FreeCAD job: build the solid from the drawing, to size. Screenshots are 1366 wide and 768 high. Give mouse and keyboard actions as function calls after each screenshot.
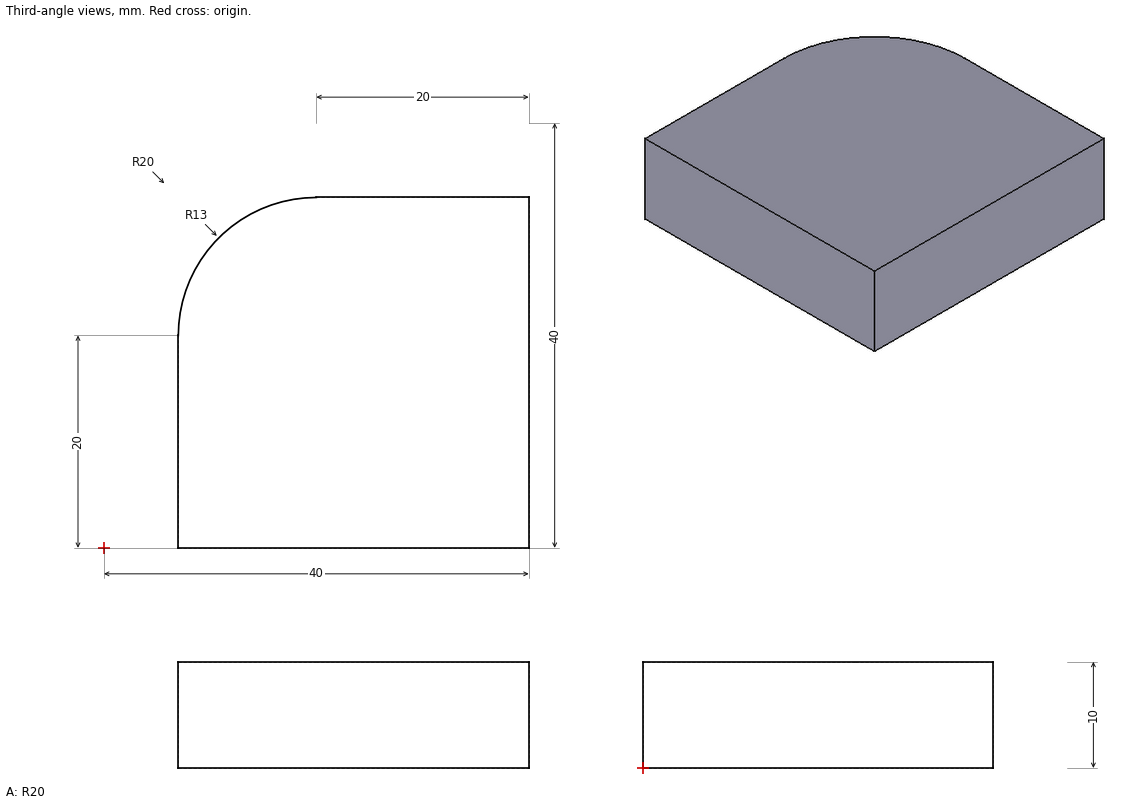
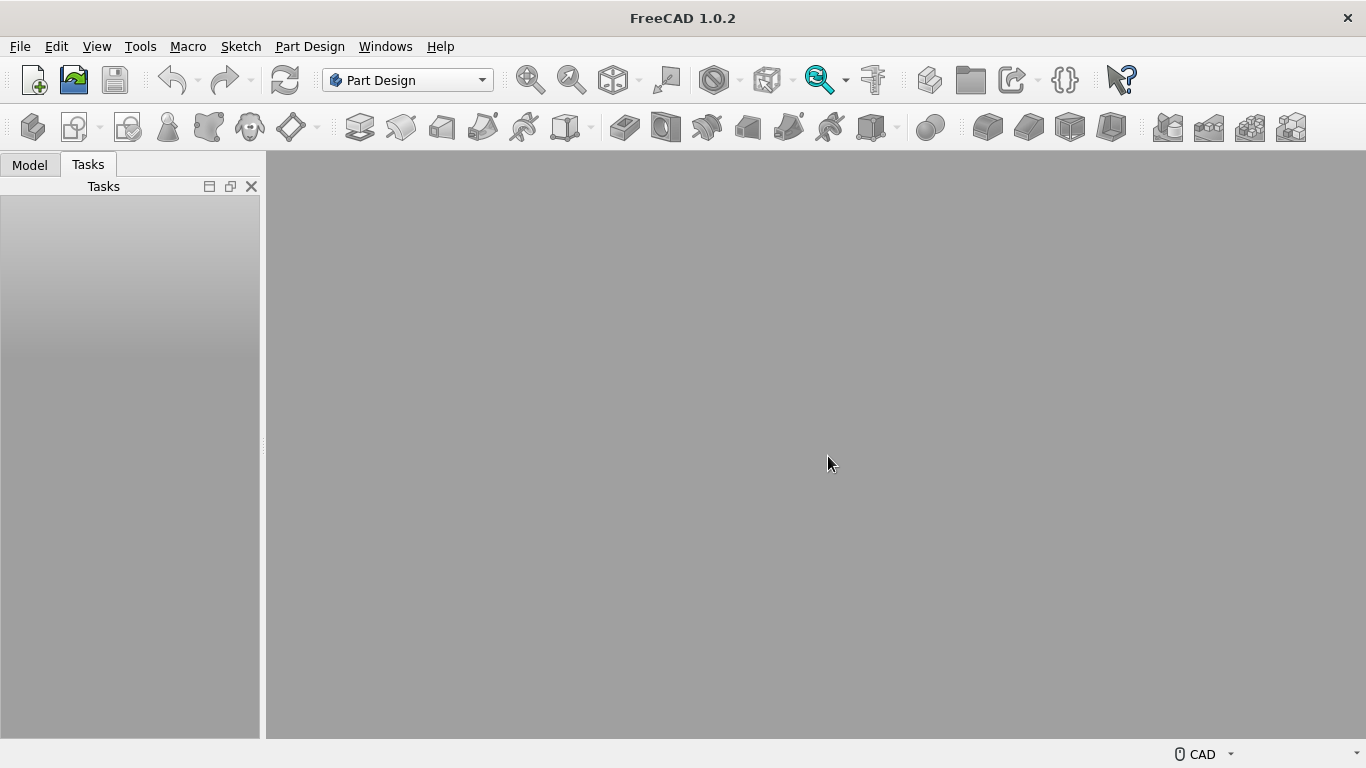
click(33, 80)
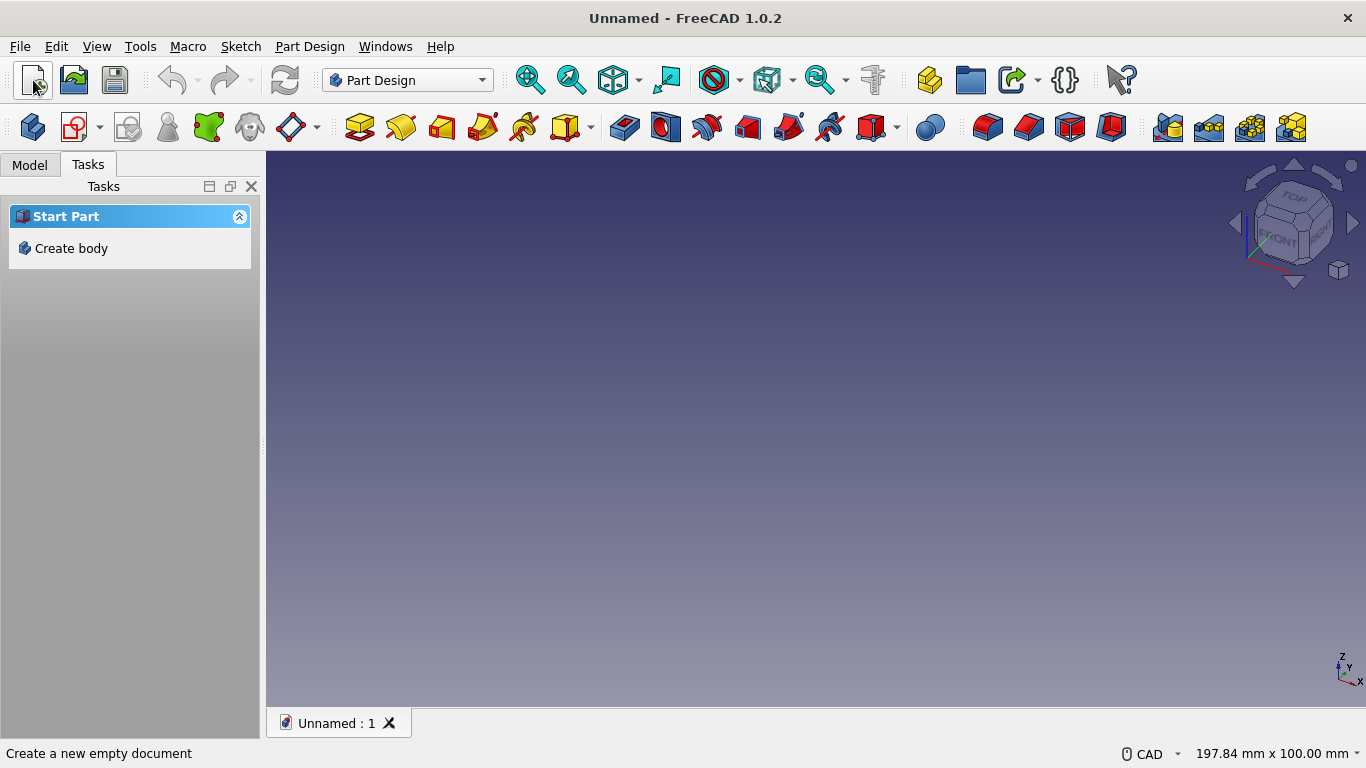
click(74, 128)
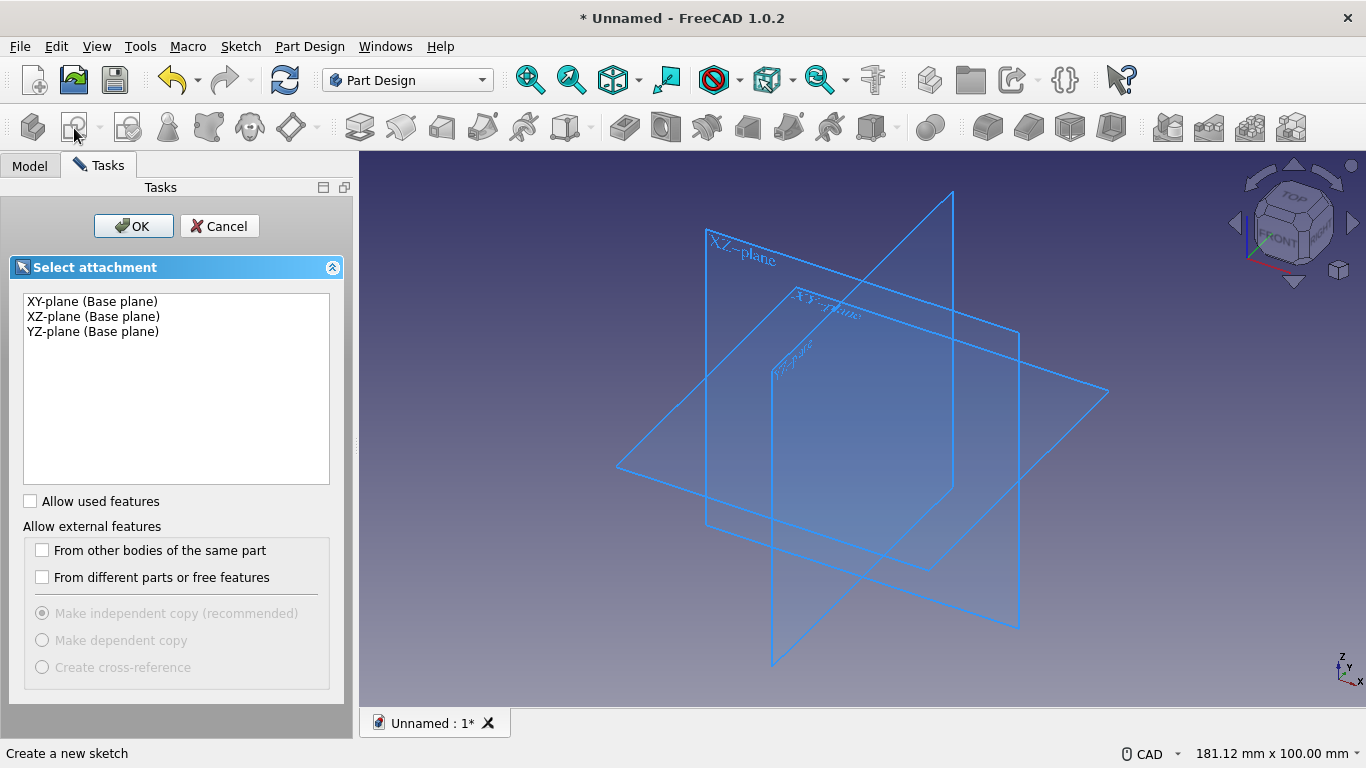
click(84, 302)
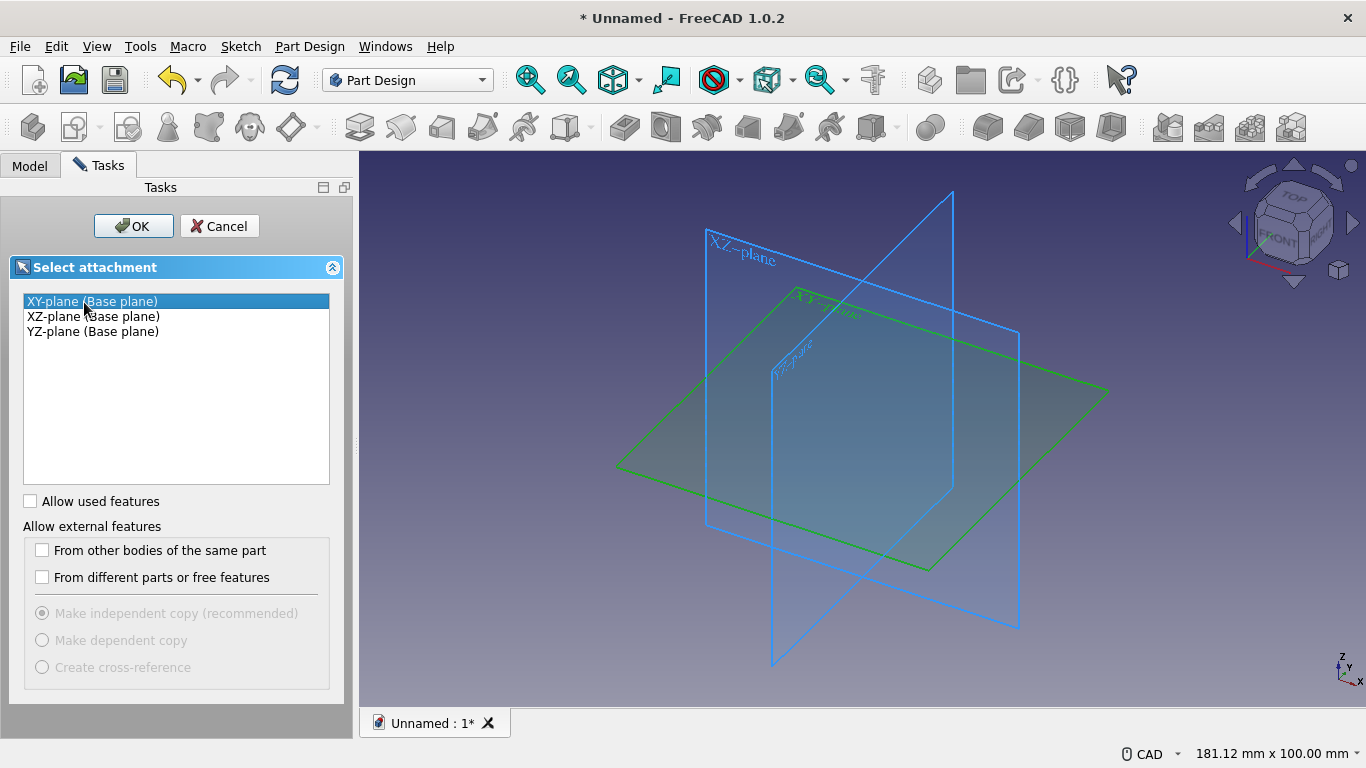
click(134, 226)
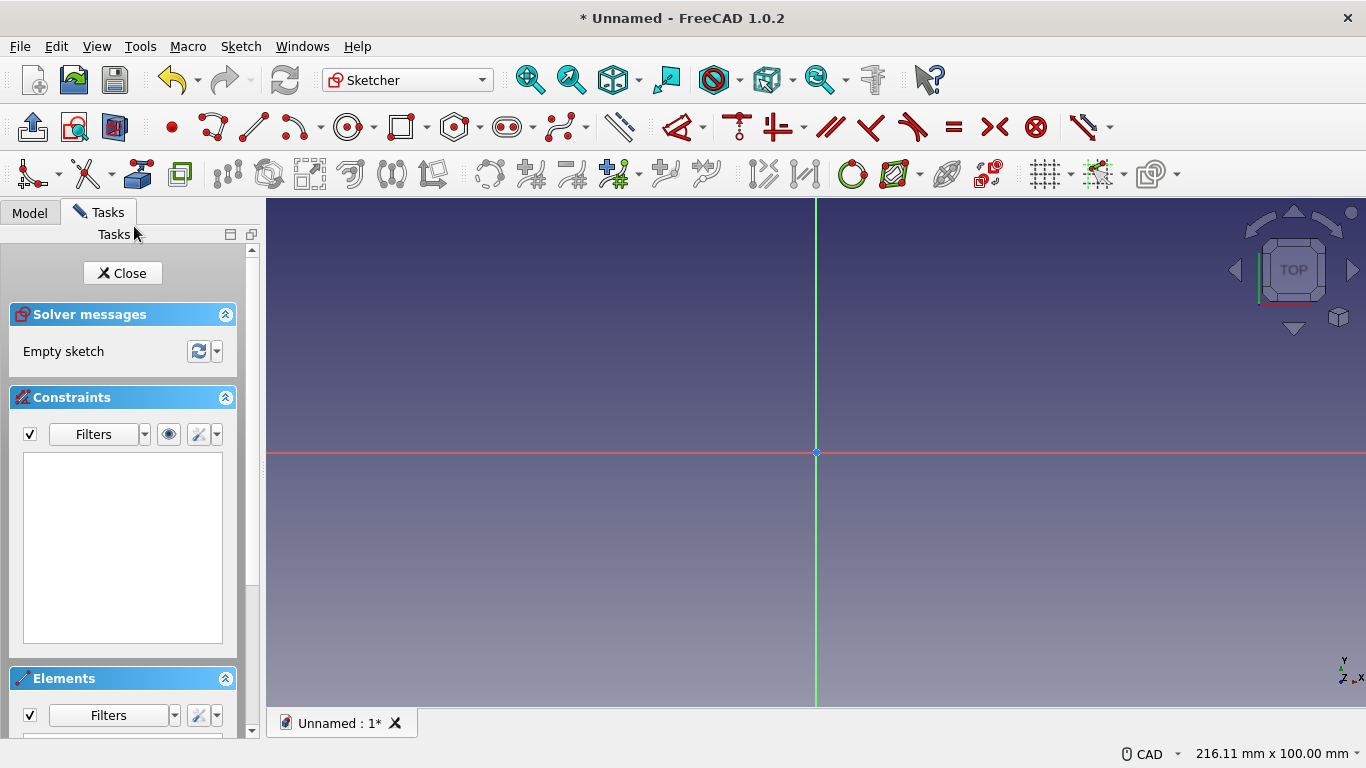
scroll(1201, 226, up, 2)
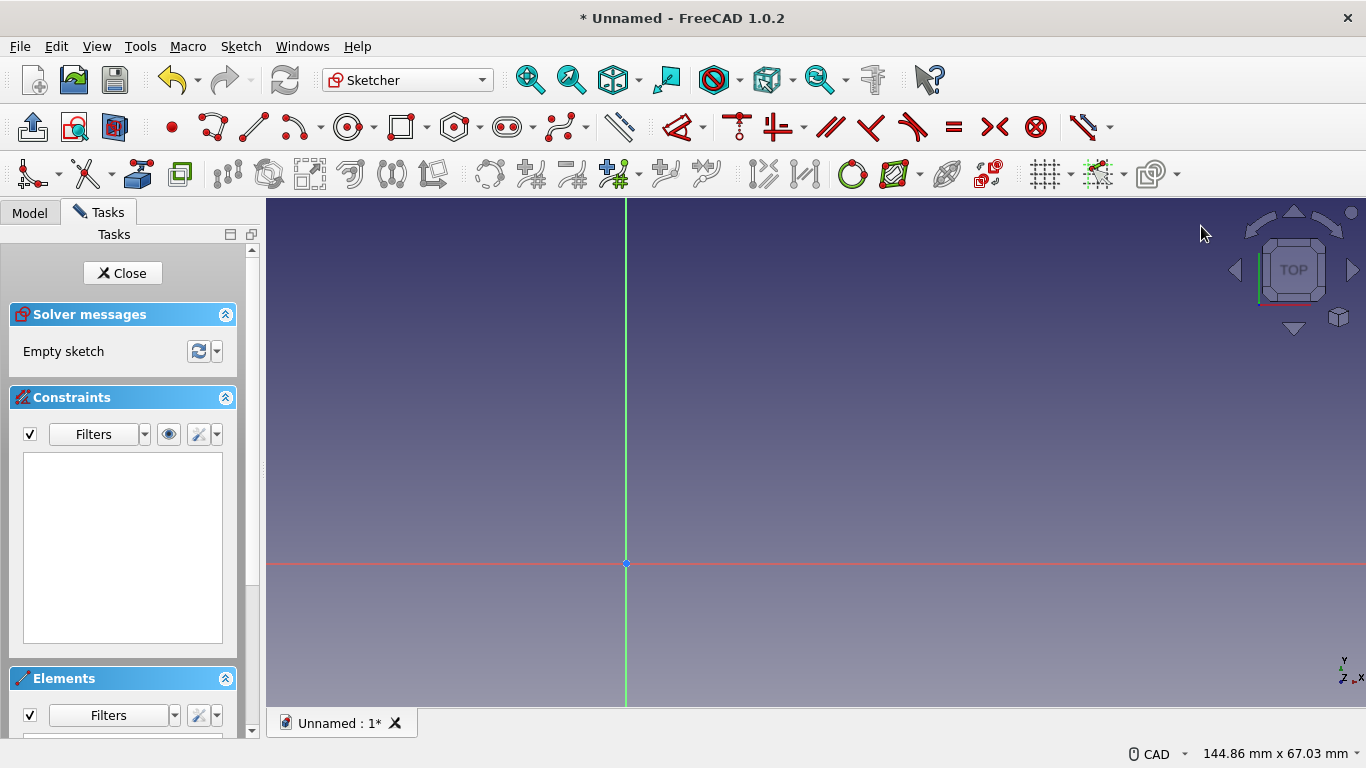
key(g)
key(r)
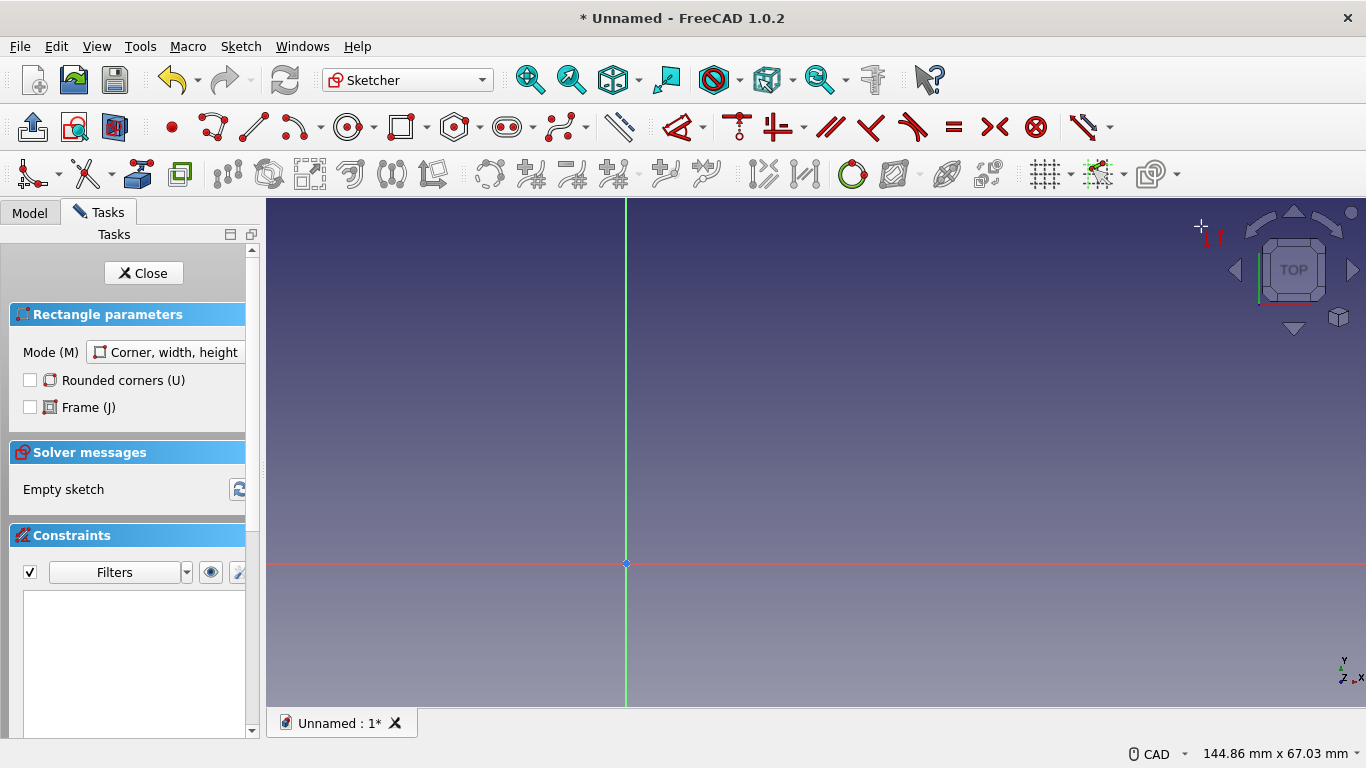
click(626, 564)
move(930, 260)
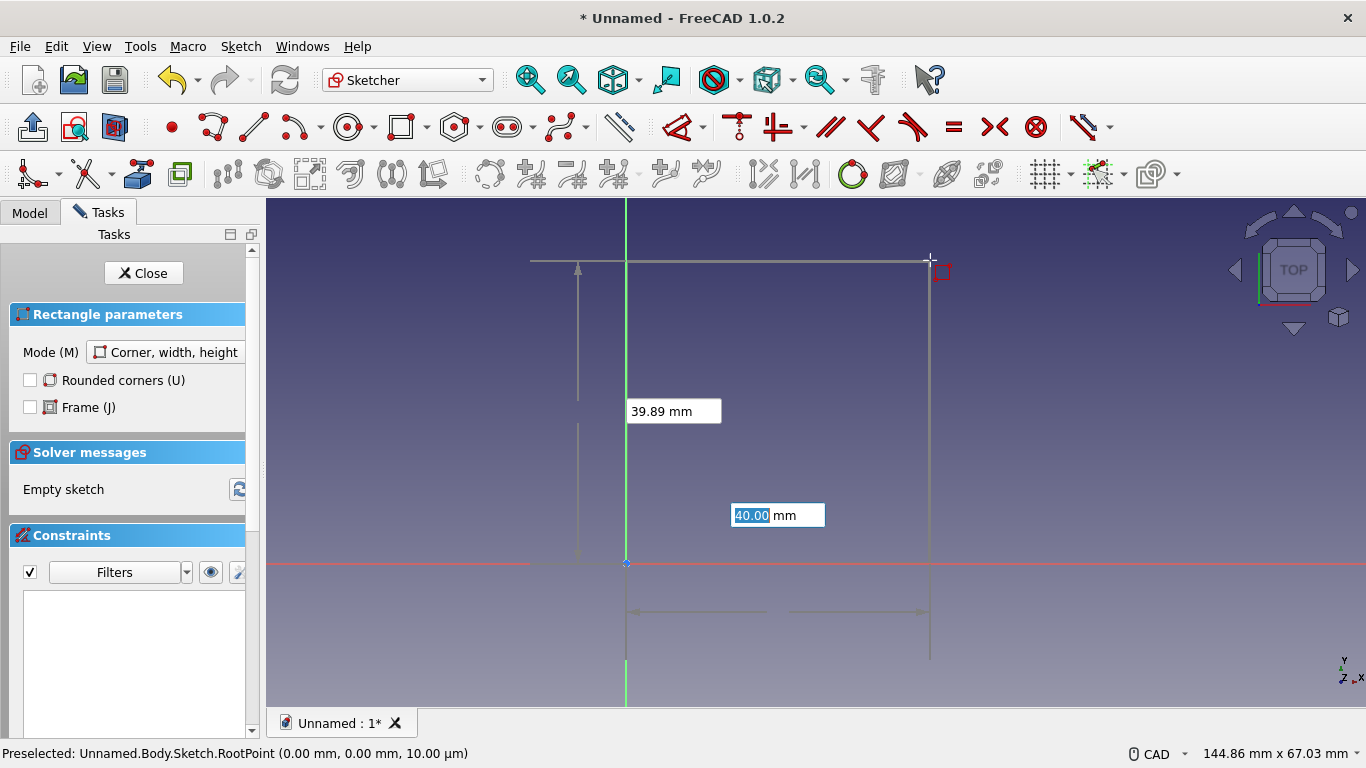
text(40)
key(Tab)
text(40)
key(Return)
key(Escape)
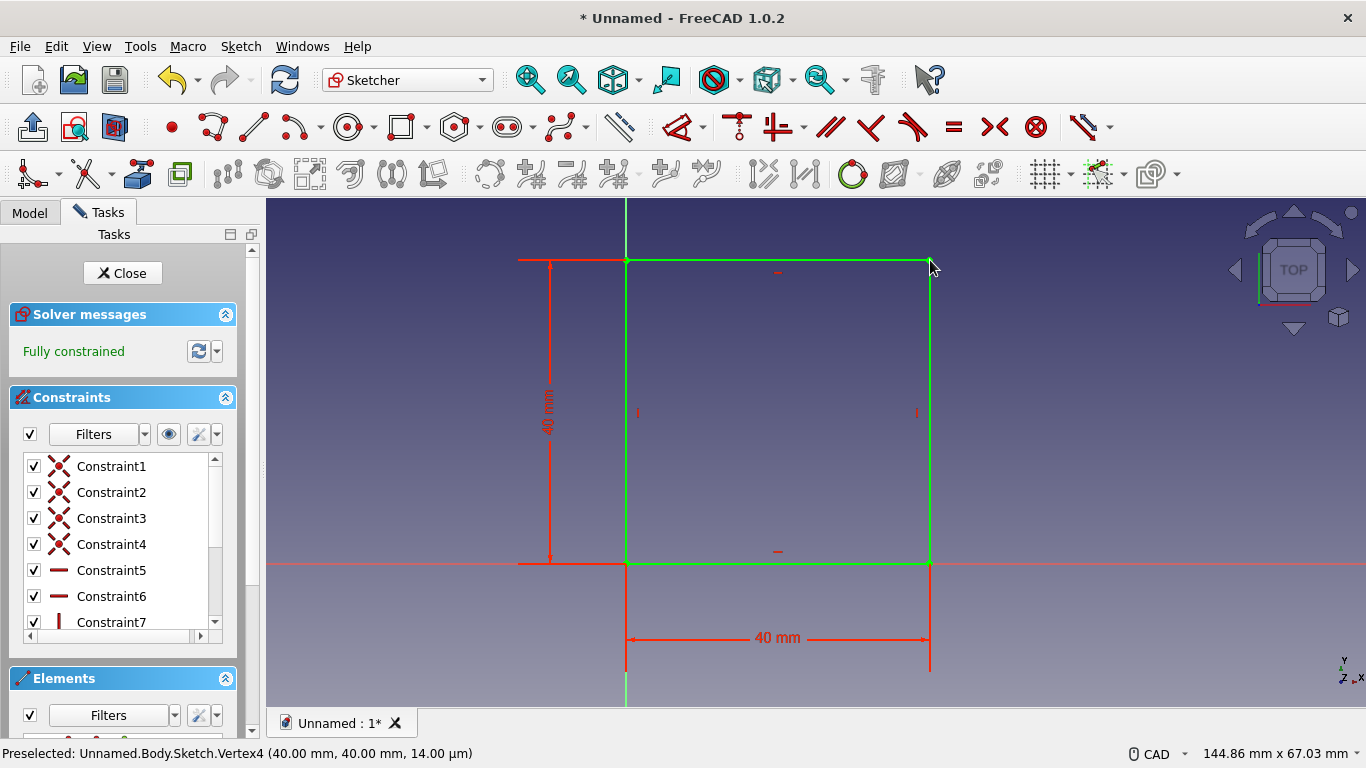
click(123, 273)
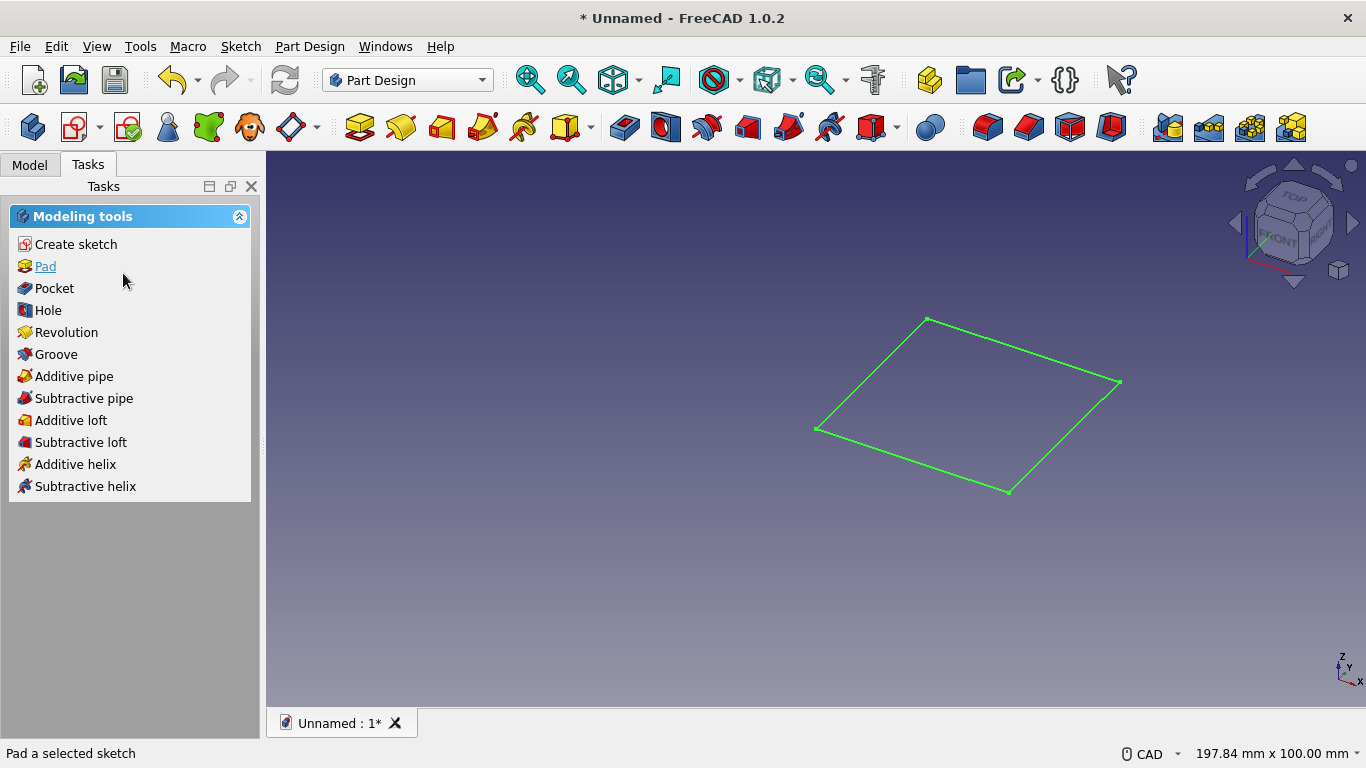
click(360, 128)